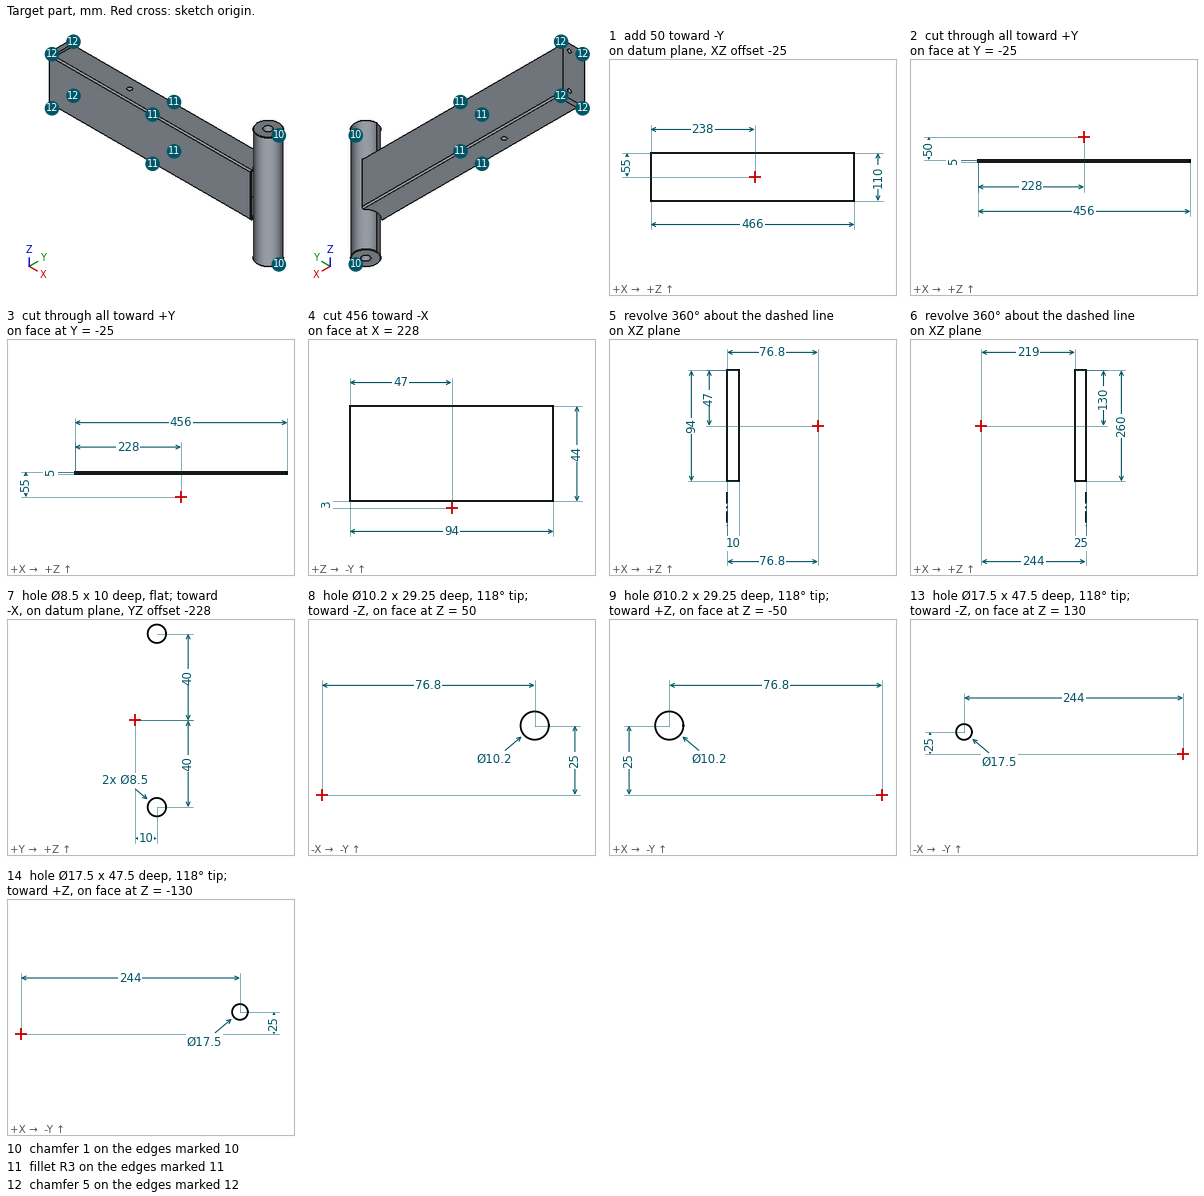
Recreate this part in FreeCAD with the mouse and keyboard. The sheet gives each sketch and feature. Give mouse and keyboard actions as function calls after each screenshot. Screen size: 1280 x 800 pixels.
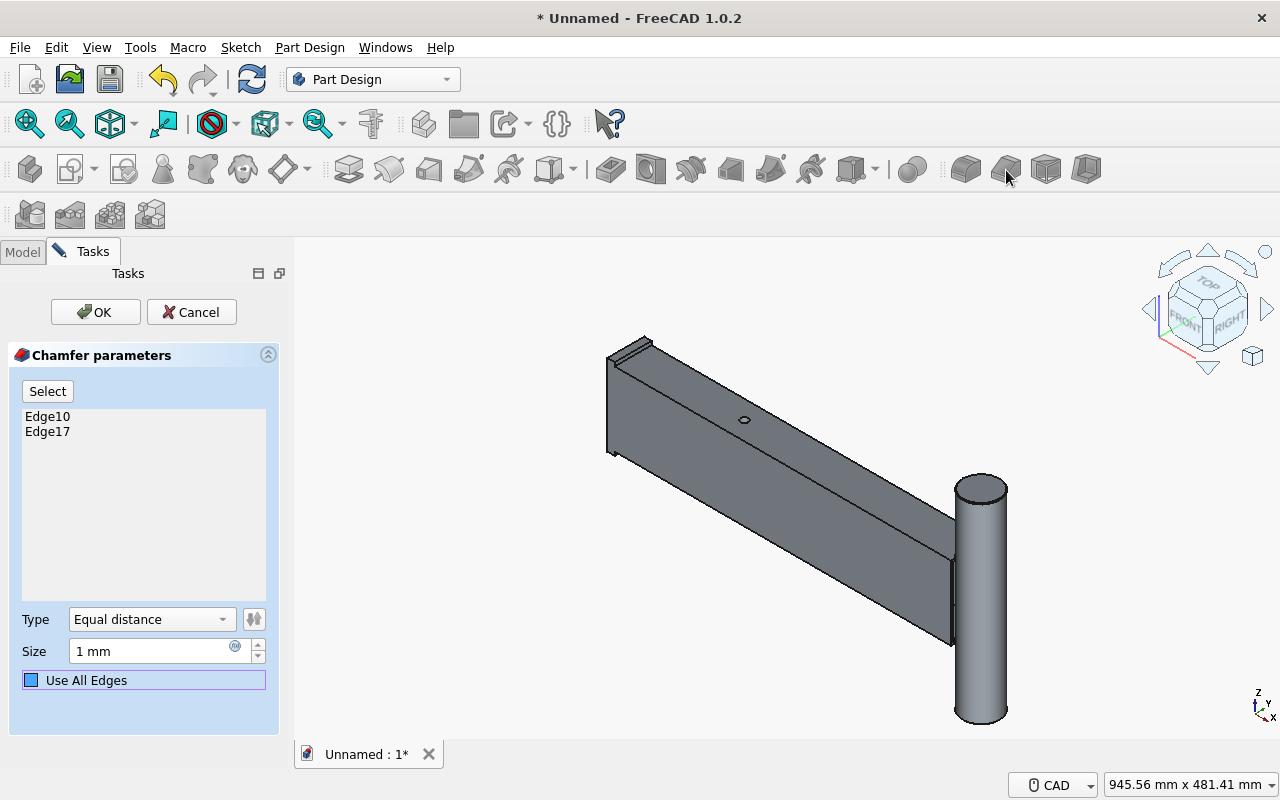
click(96, 312)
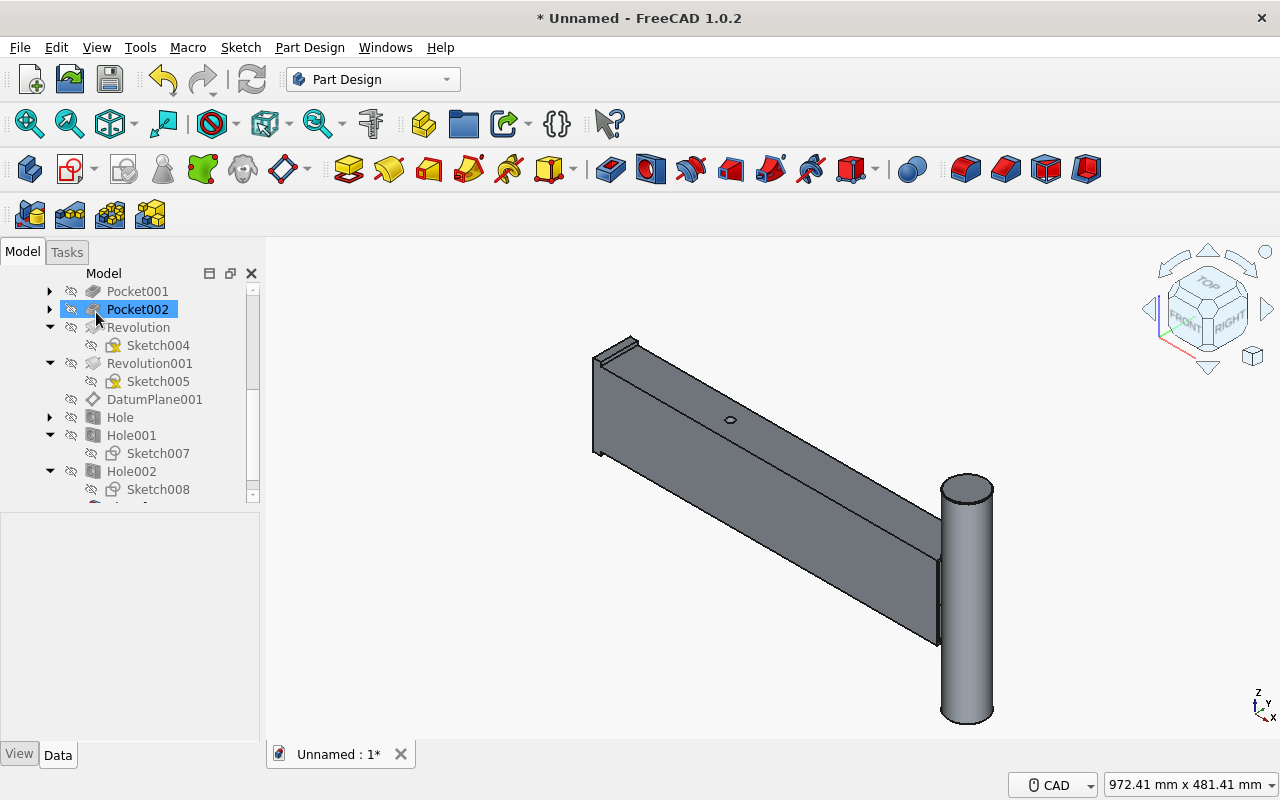
click(769, 463)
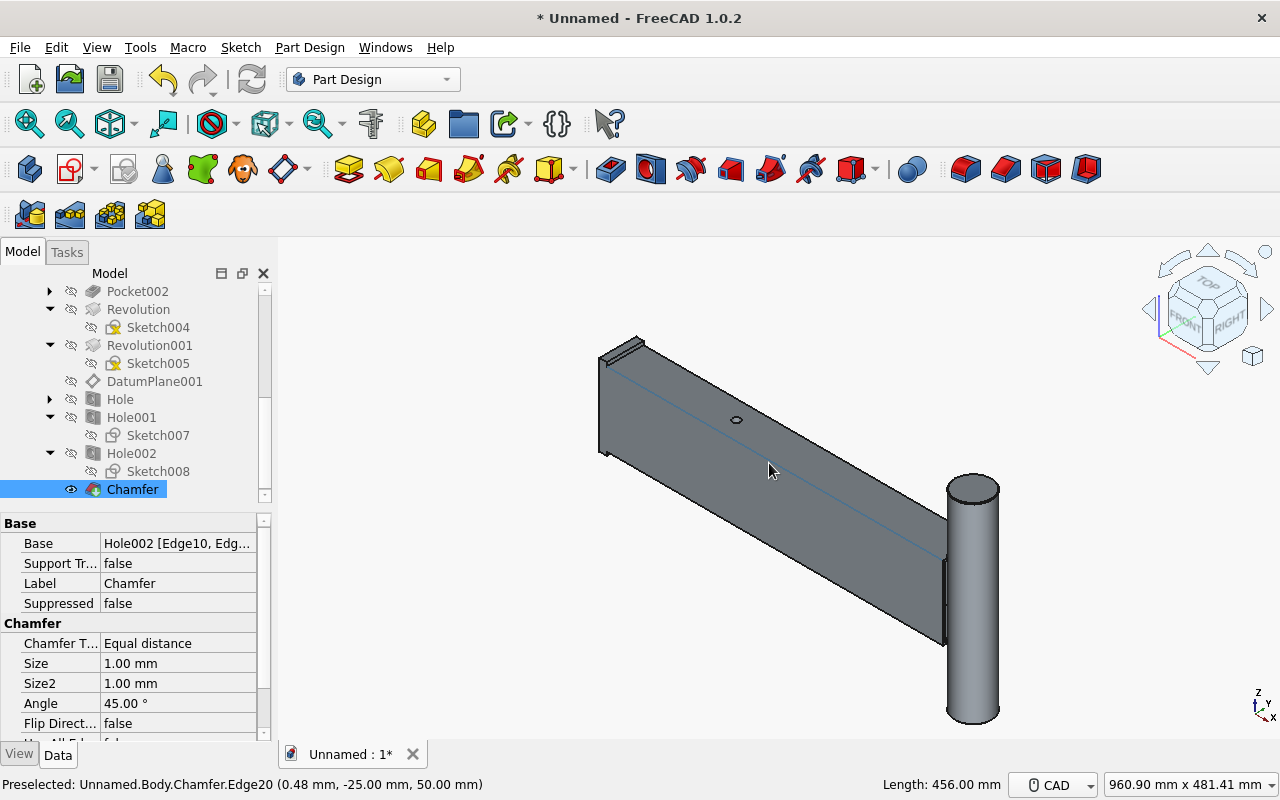
key(2)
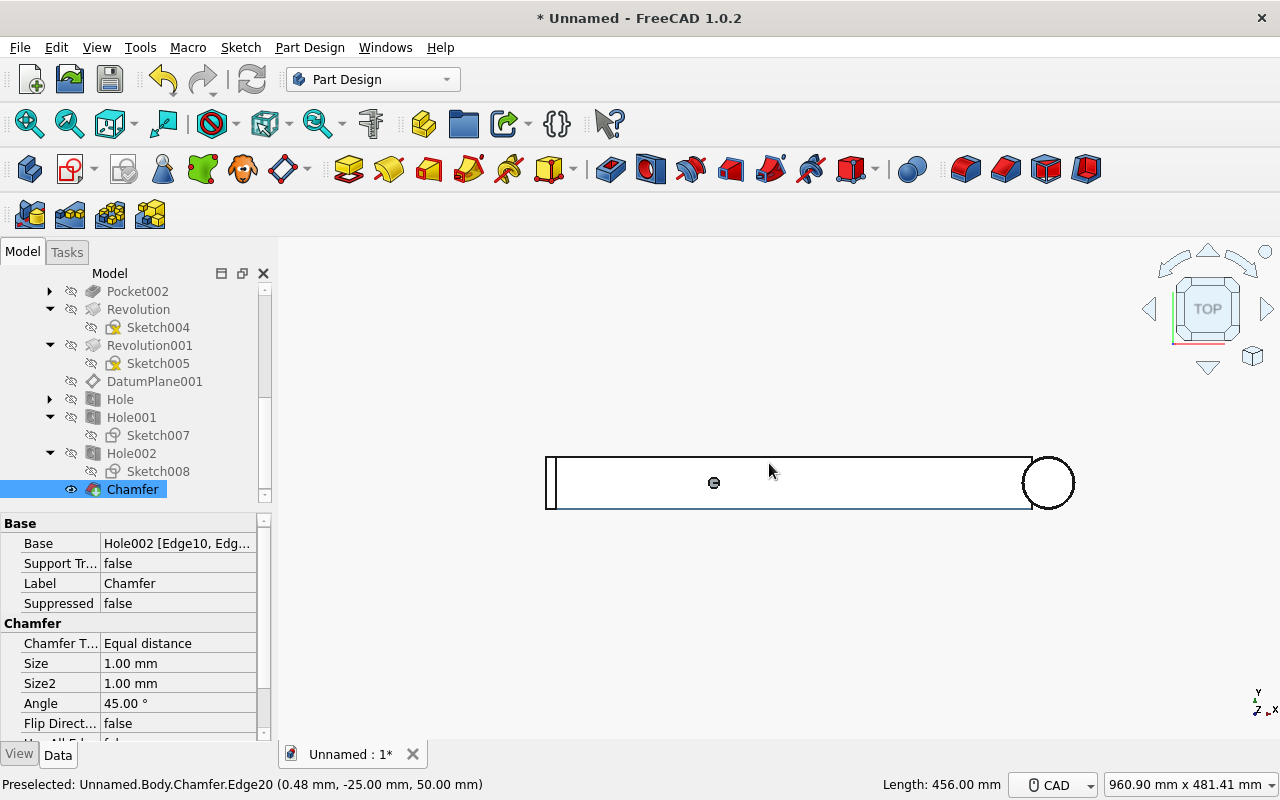
click(794, 456, ctrl)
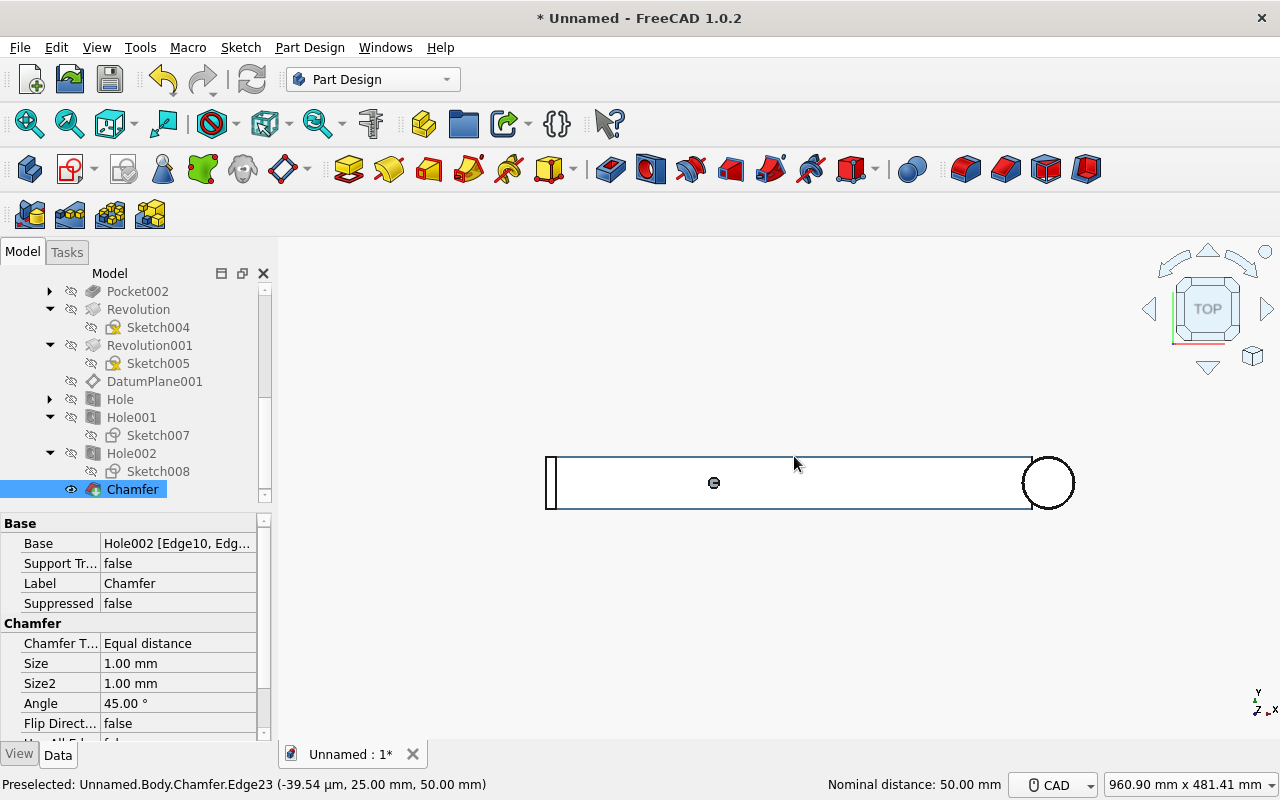
key(0)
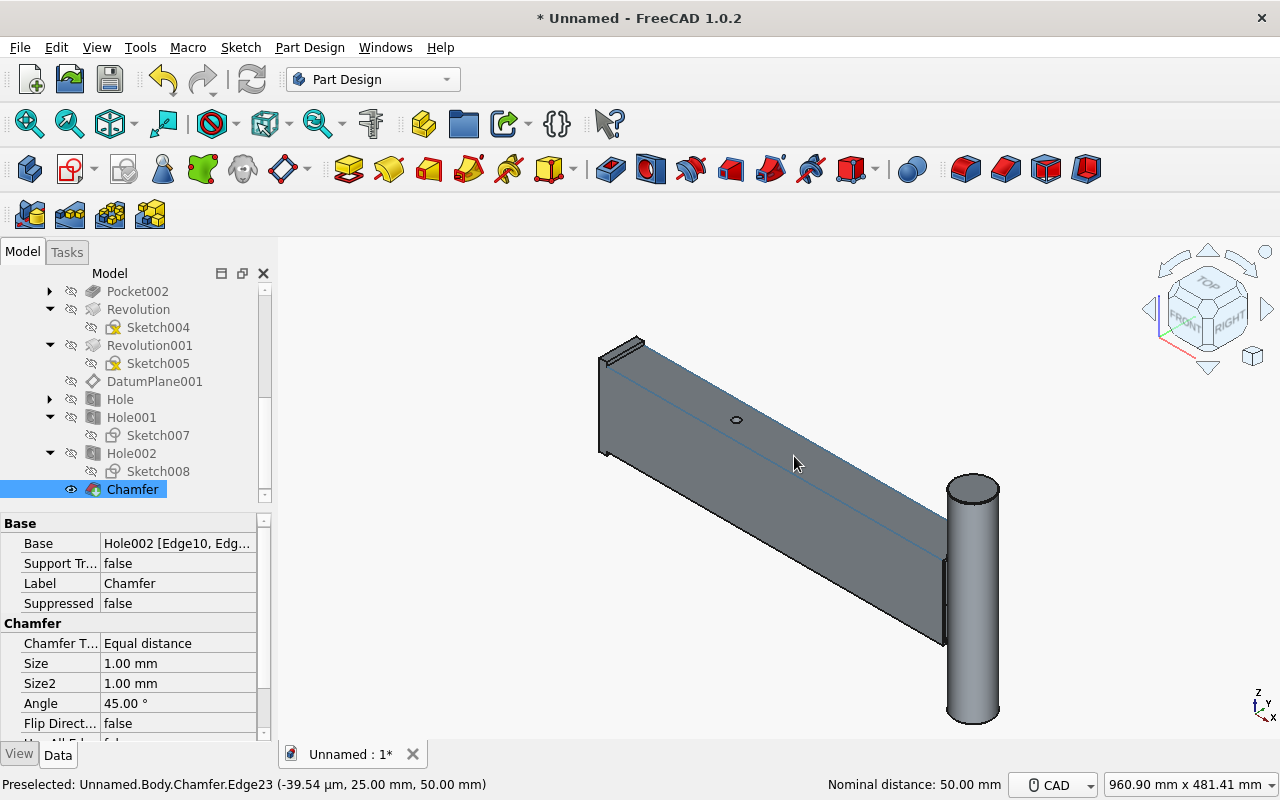
key(1)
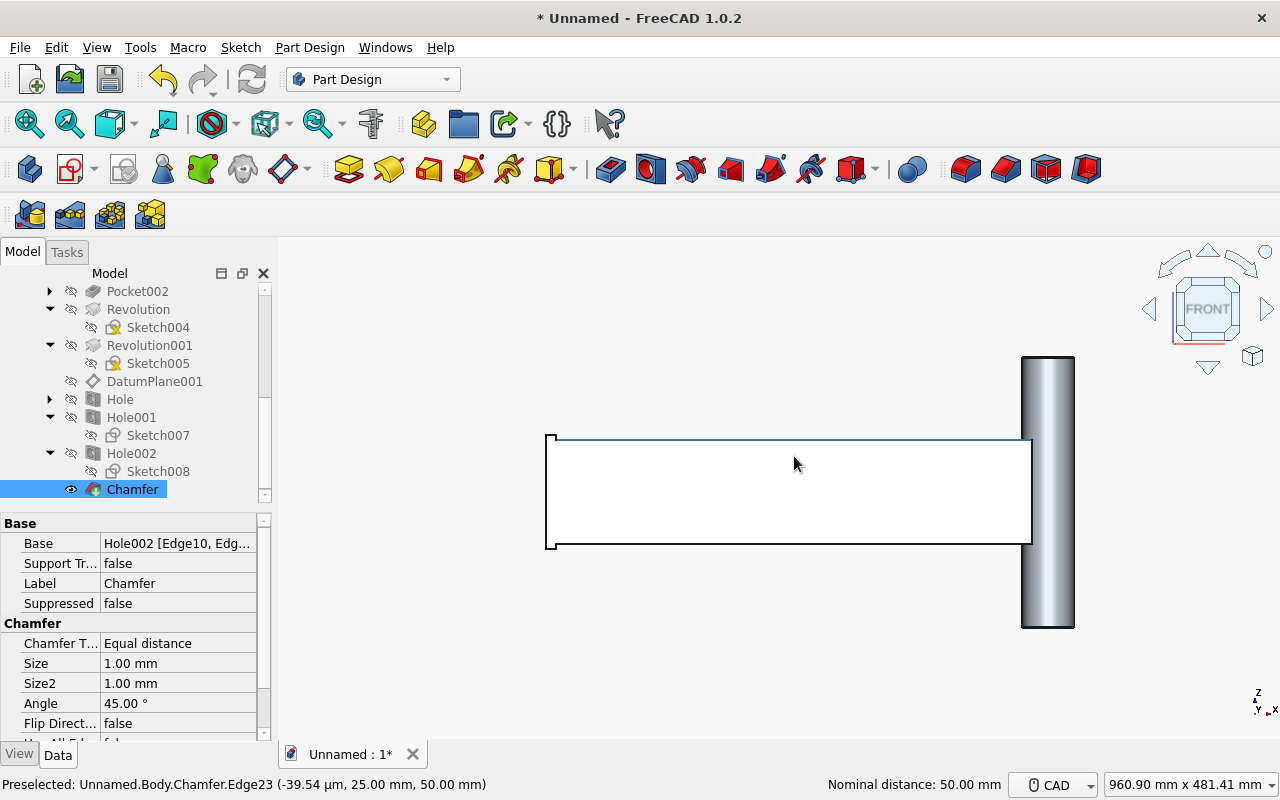
key(3)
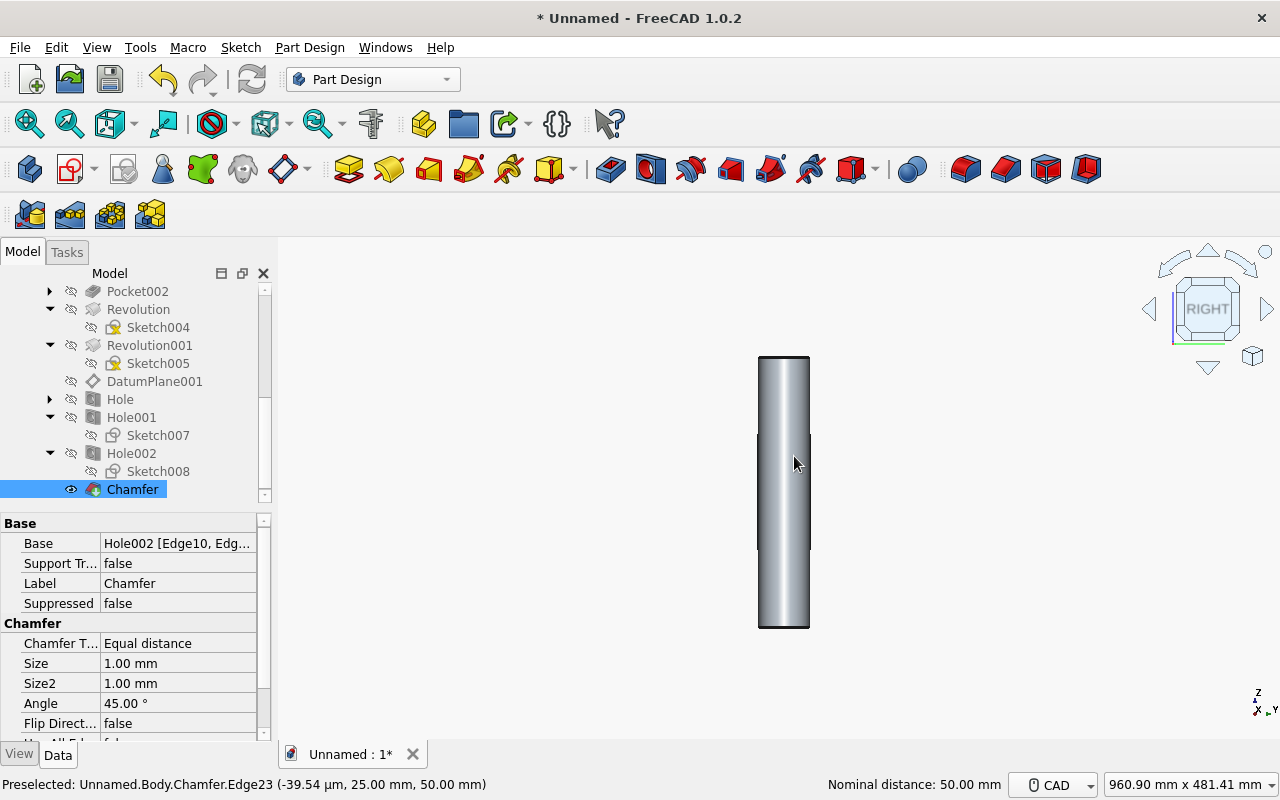
key(5)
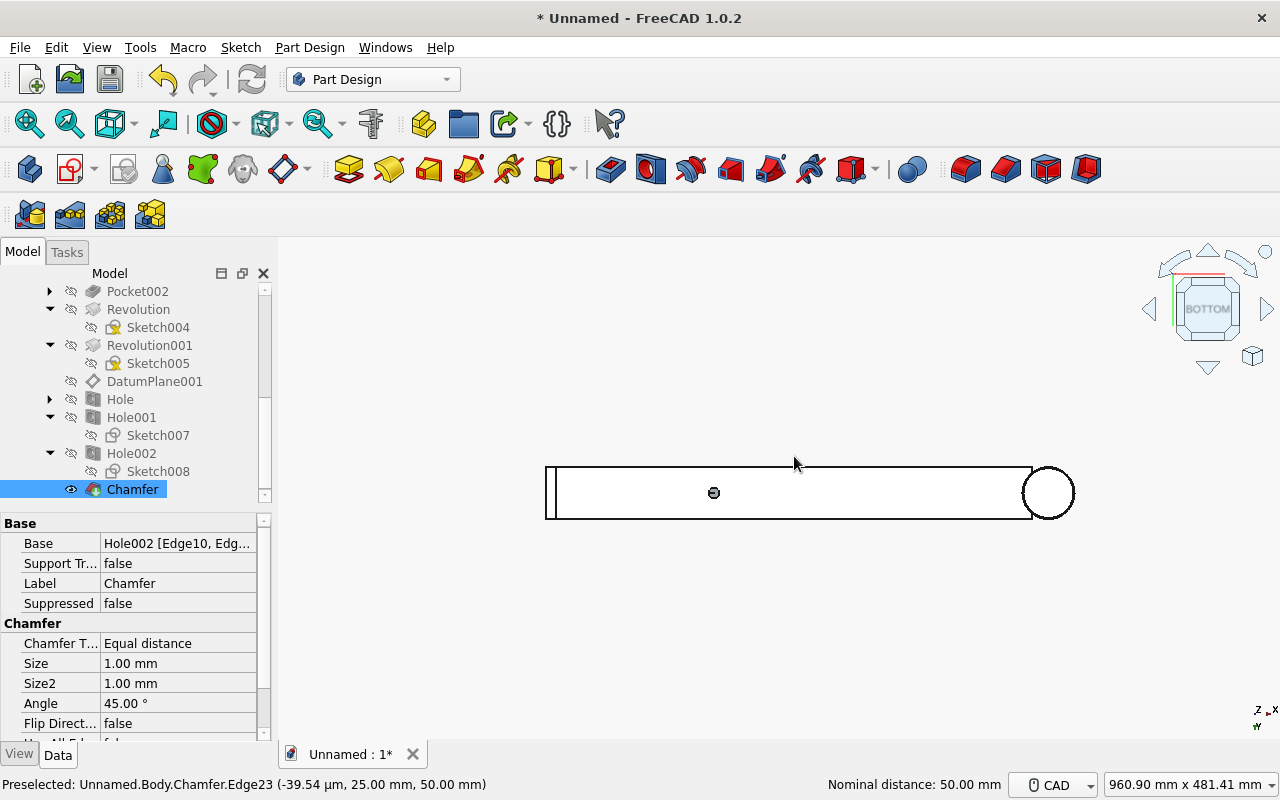
click(794, 466, ctrl)